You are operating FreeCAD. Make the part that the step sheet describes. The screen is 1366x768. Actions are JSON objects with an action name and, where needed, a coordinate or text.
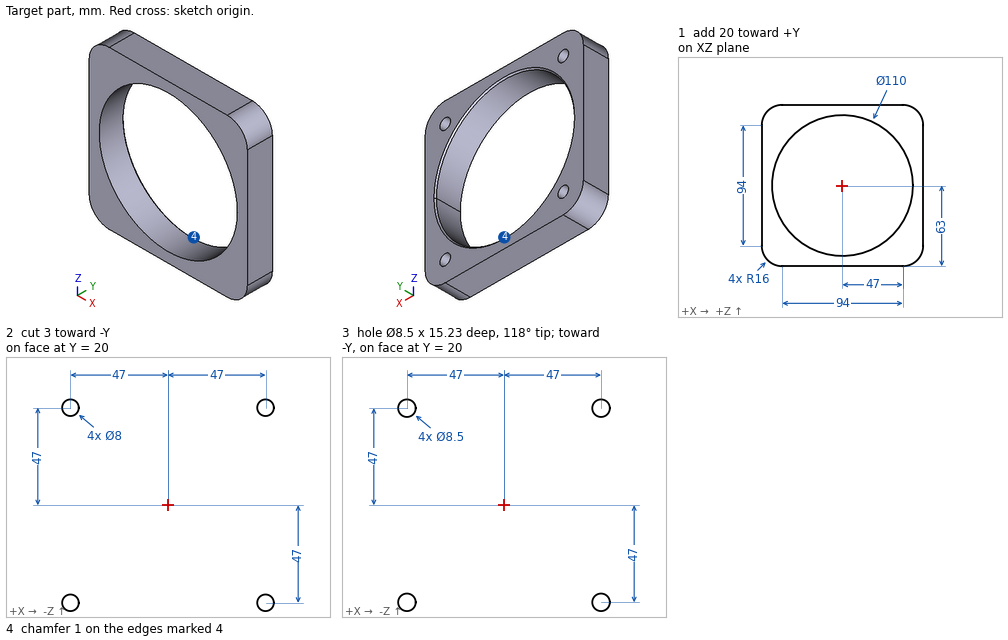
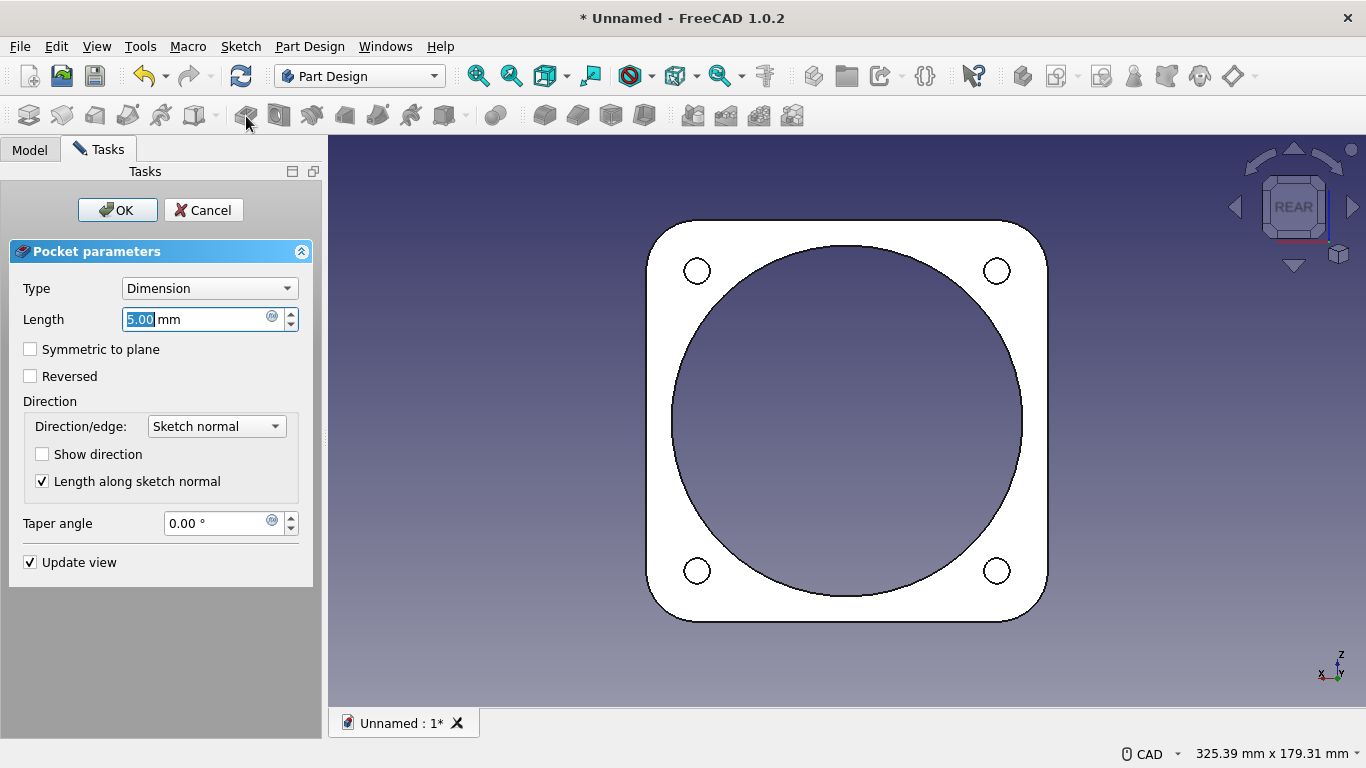
{"action": "type", "text": "3"}
{"action": "key", "text": "Tab"}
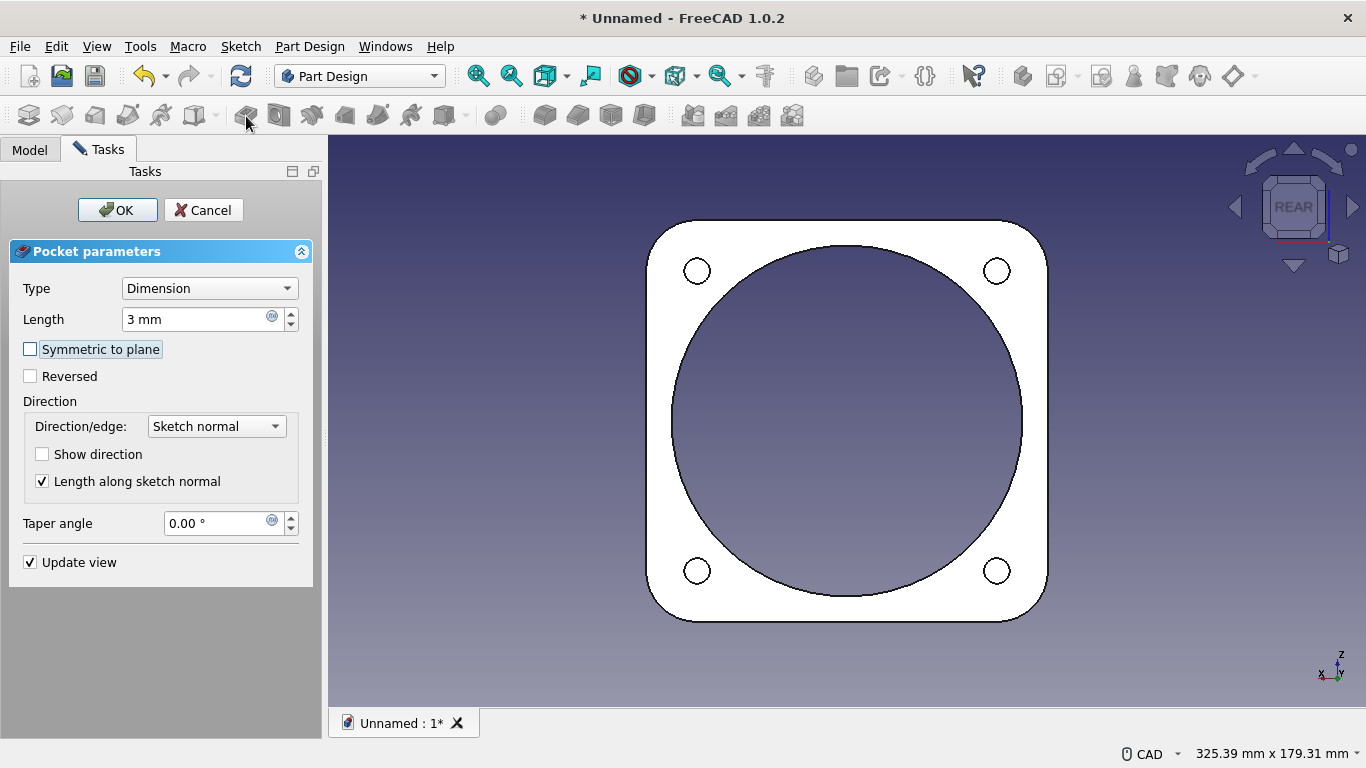
{"action": "left_click", "coordinate": [118, 210]}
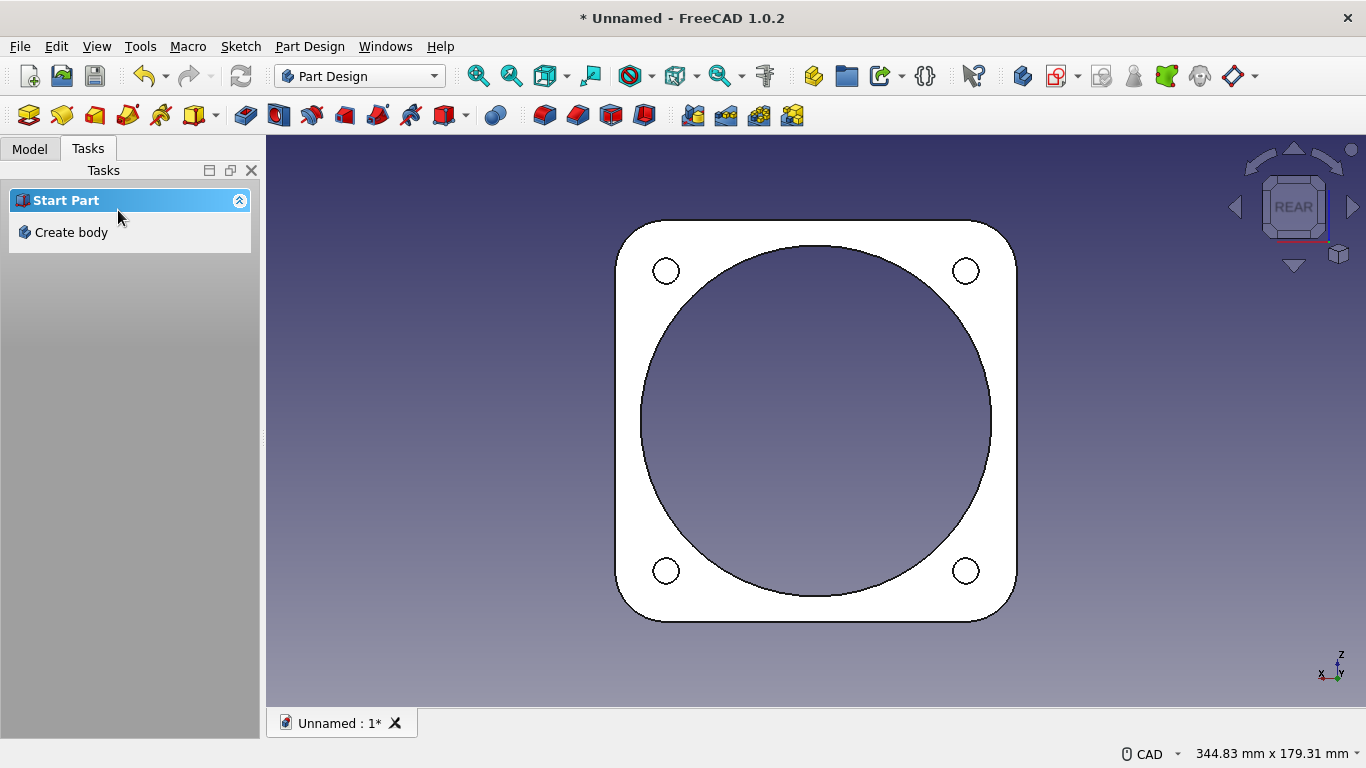
{"action": "left_click", "coordinate": [644, 305]}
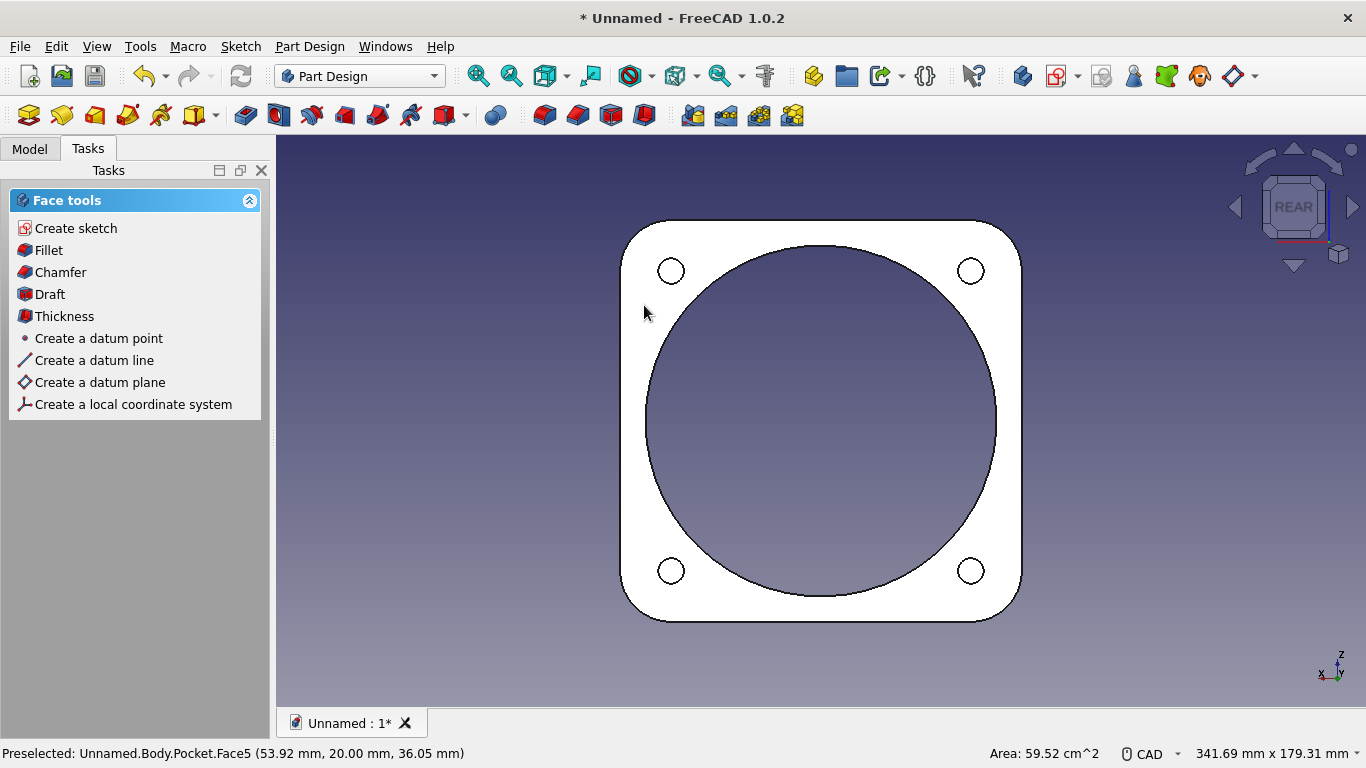
{"action": "left_click", "coordinate": [1056, 76]}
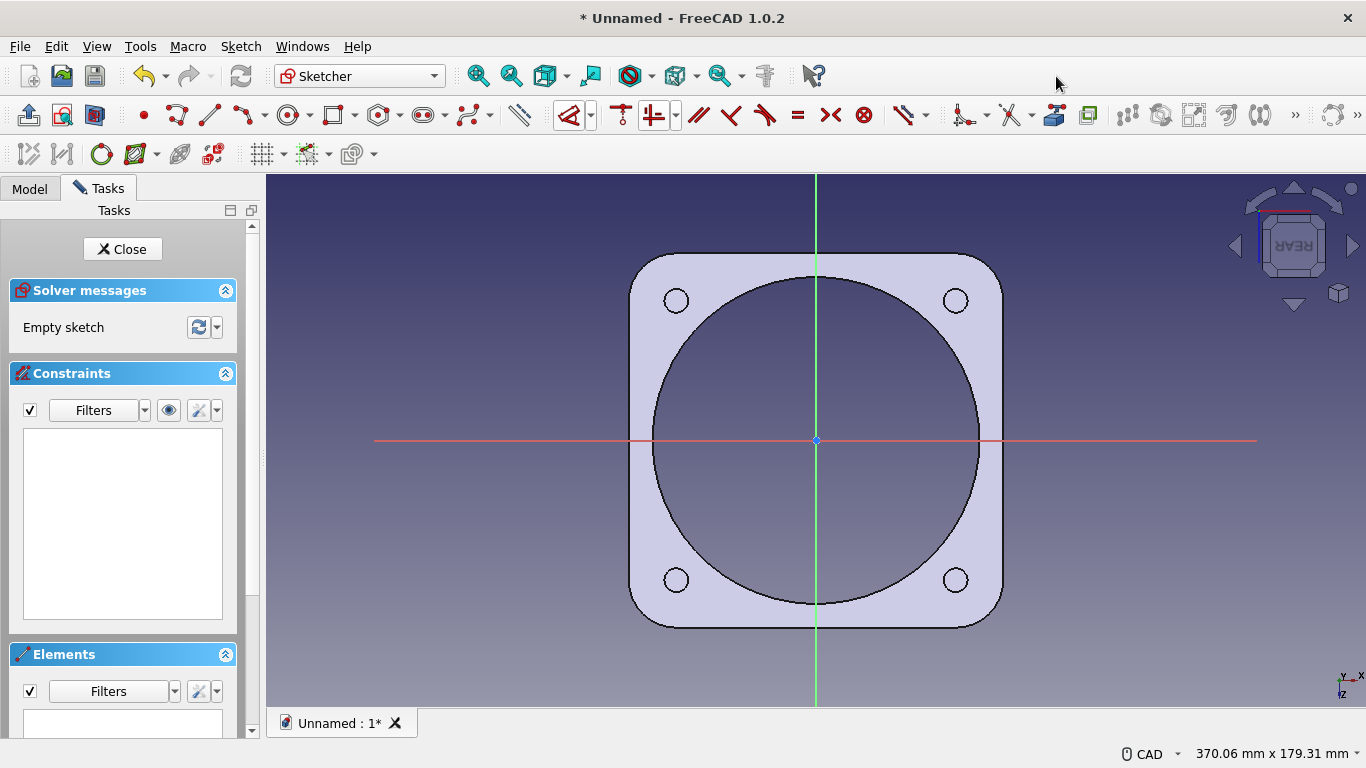
{"action": "left_click", "coordinate": [288, 116]}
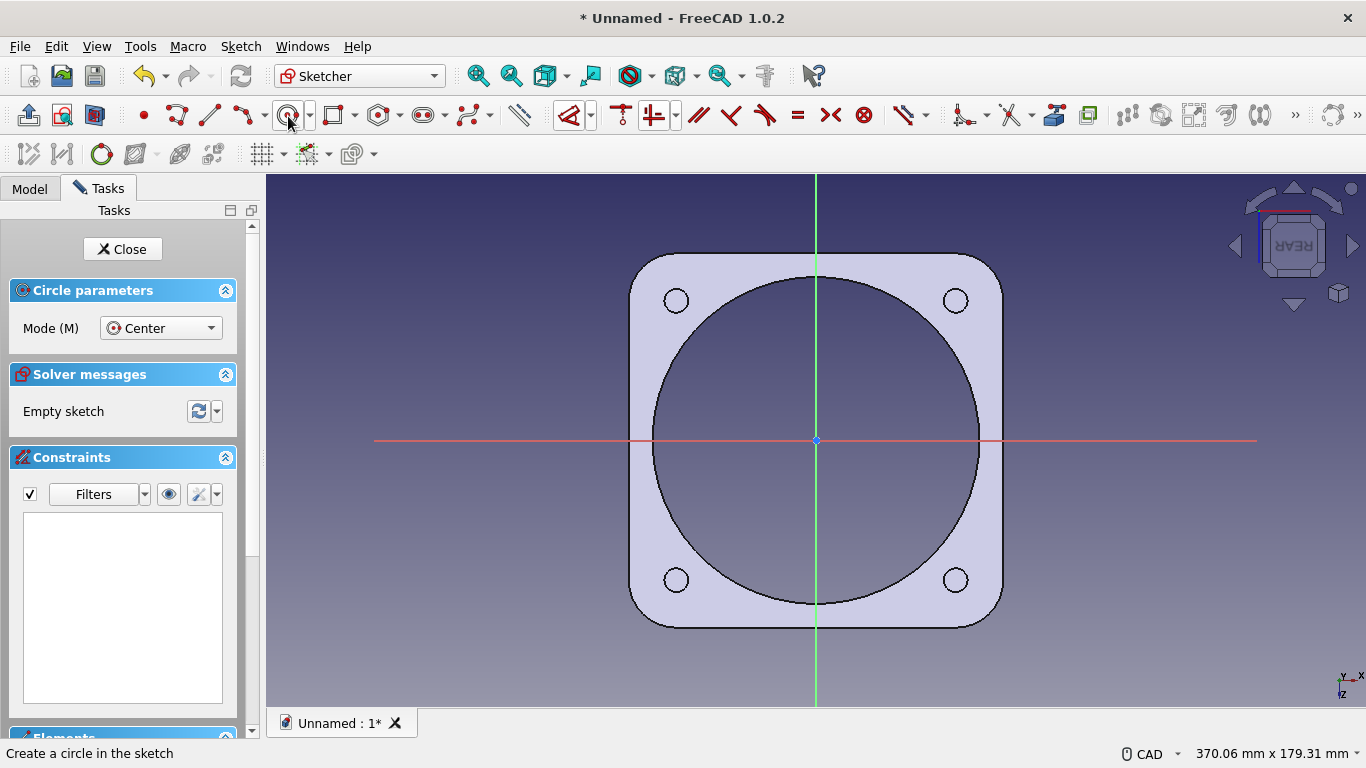
{"action": "scroll", "coordinate": [676, 301], "scroll_direction": "up", "scroll_amount": 3}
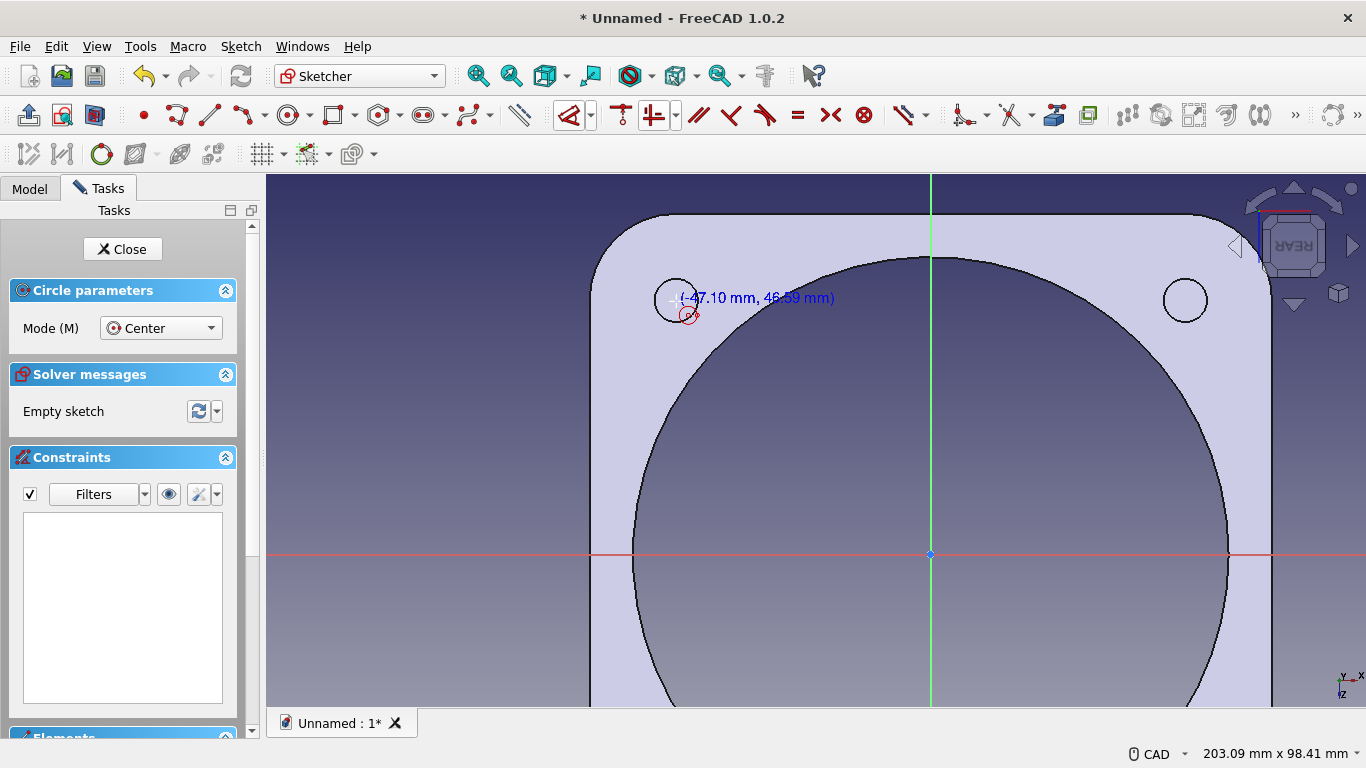
{"action": "left_click", "coordinate": [676, 300]}
{"action": "left_click", "coordinate": [693, 284]}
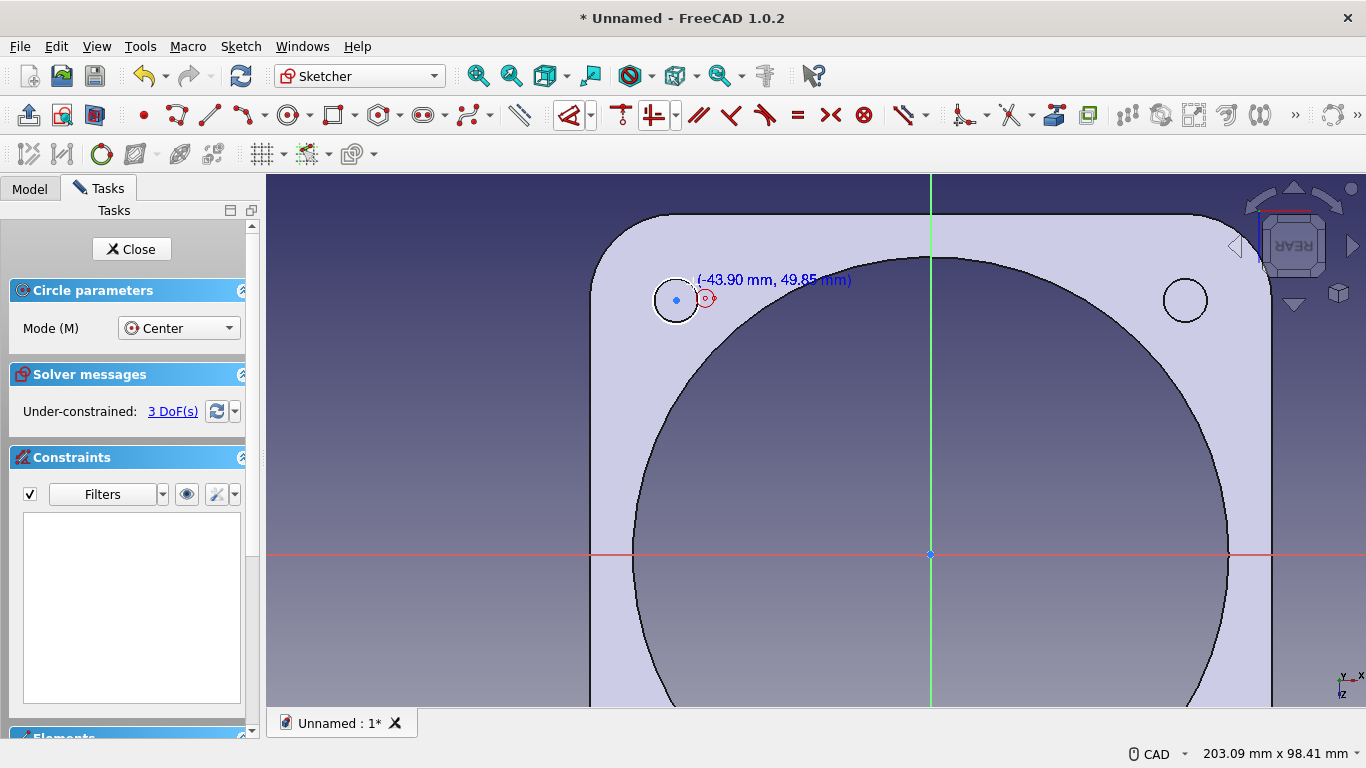
{"action": "left_click", "coordinate": [1185, 300]}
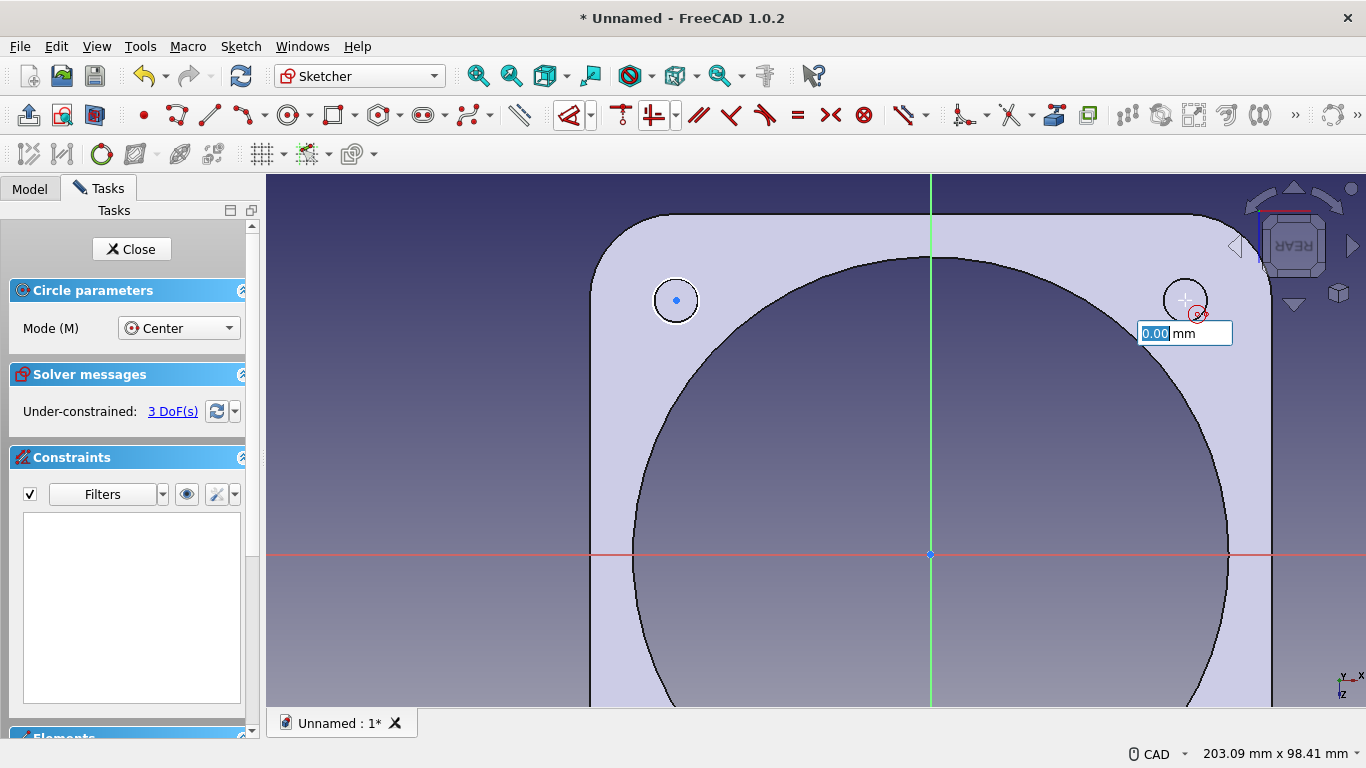
{"action": "scroll", "coordinate": [525, 301], "scroll_direction": "down", "scroll_amount": 3}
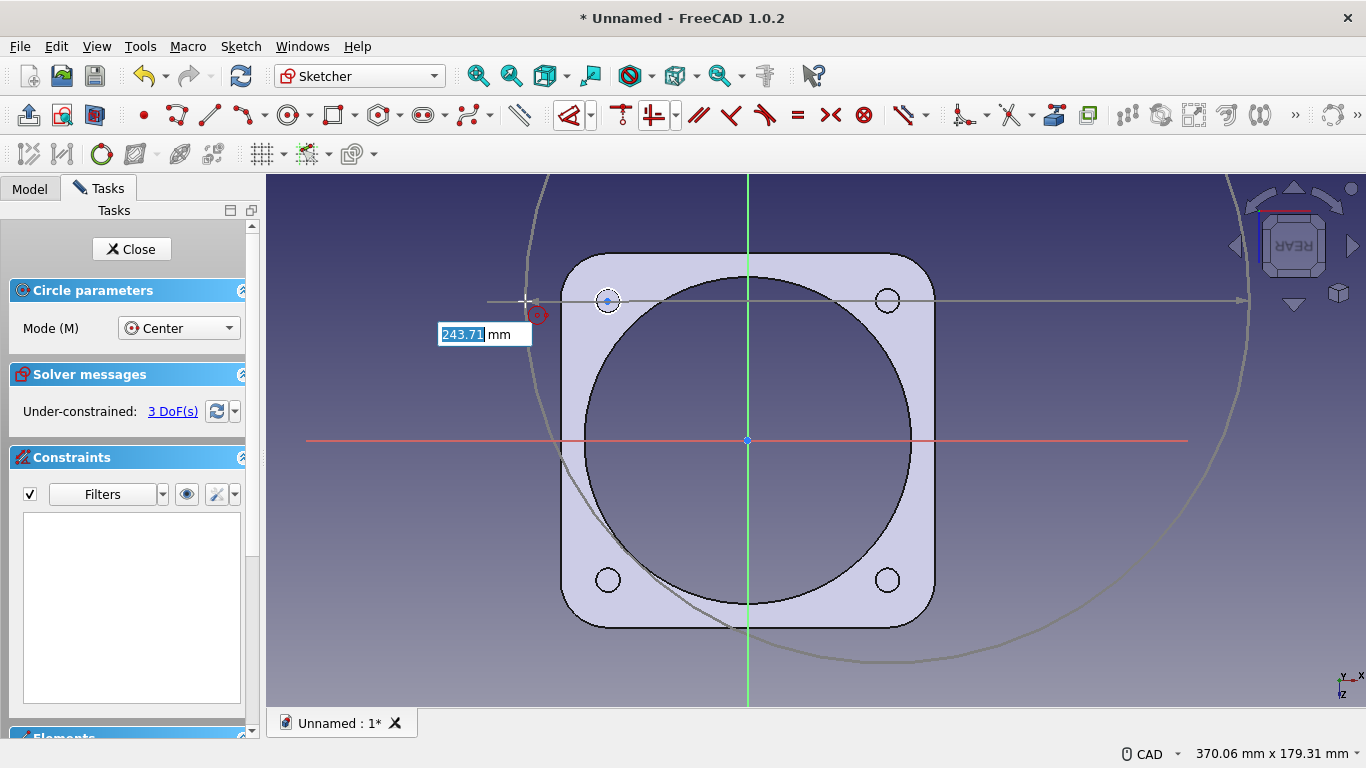
{"action": "scroll", "coordinate": [896, 292], "scroll_direction": "up", "scroll_amount": 2}